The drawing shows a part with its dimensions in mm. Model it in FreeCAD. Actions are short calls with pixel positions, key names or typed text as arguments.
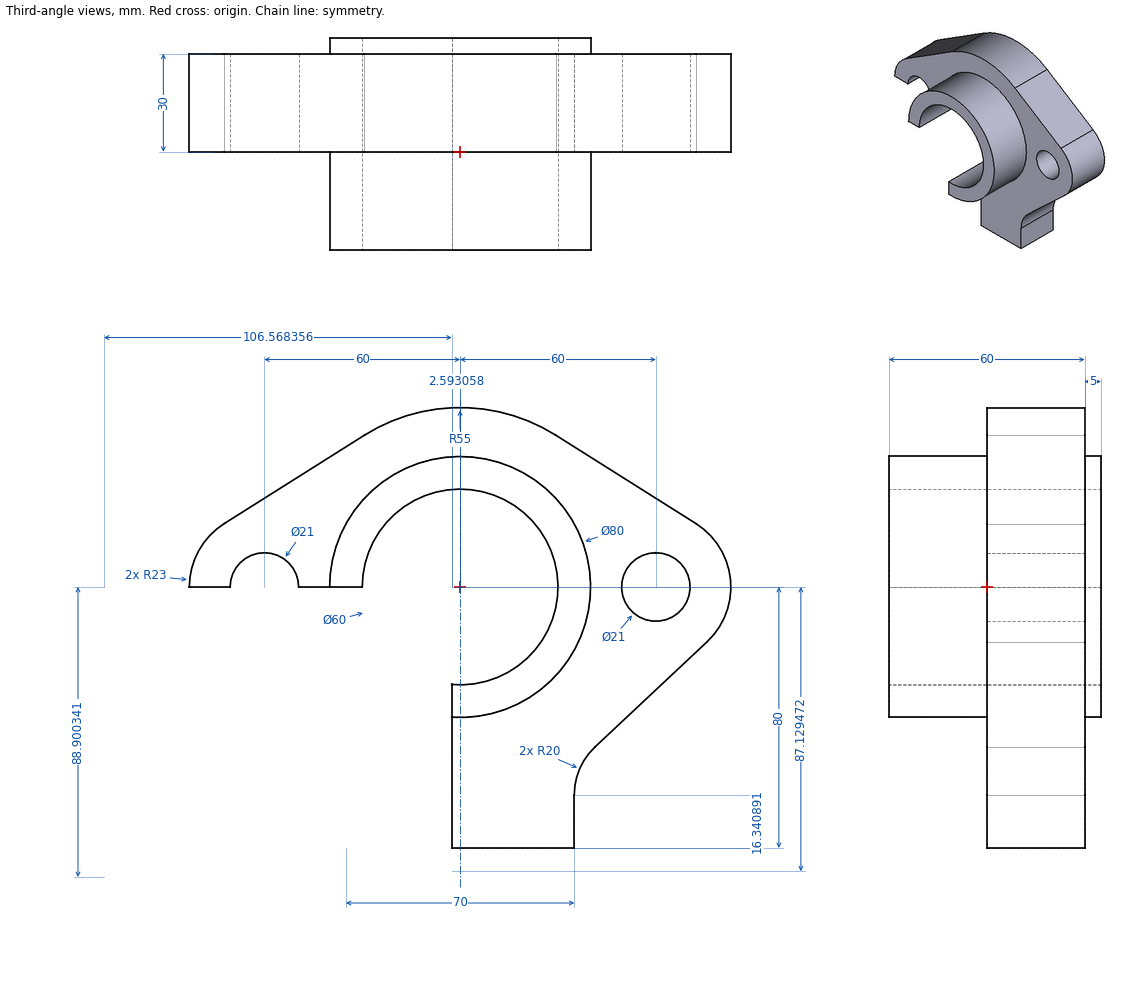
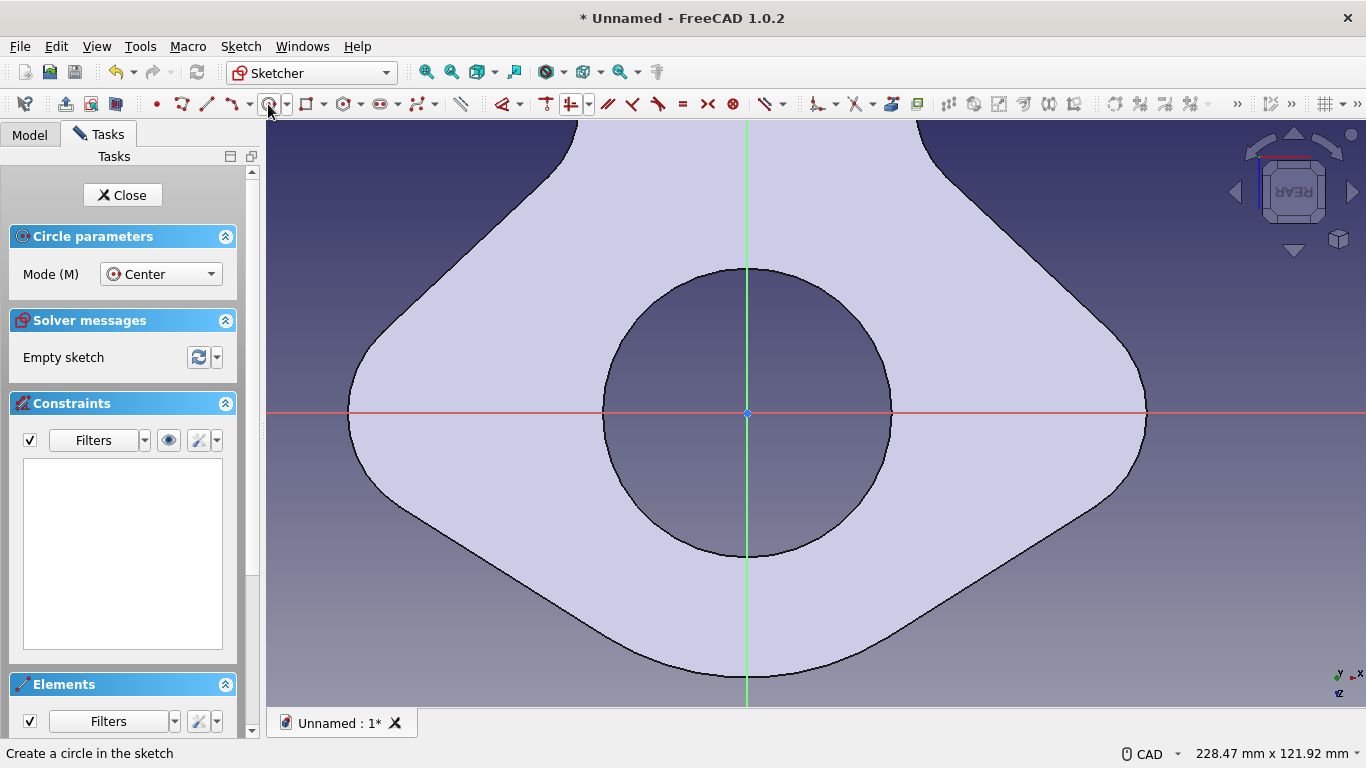
click(747, 413)
move(883, 277)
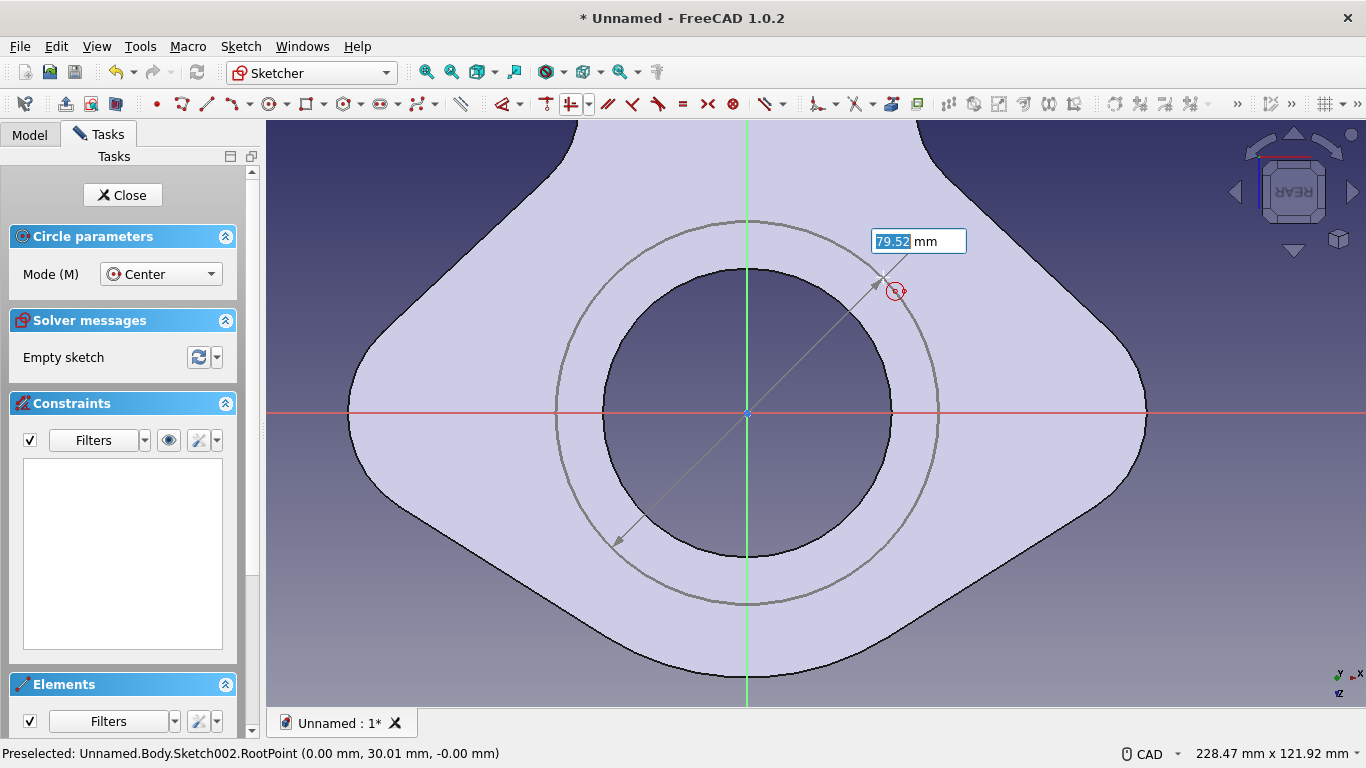
text(80)
key(Return)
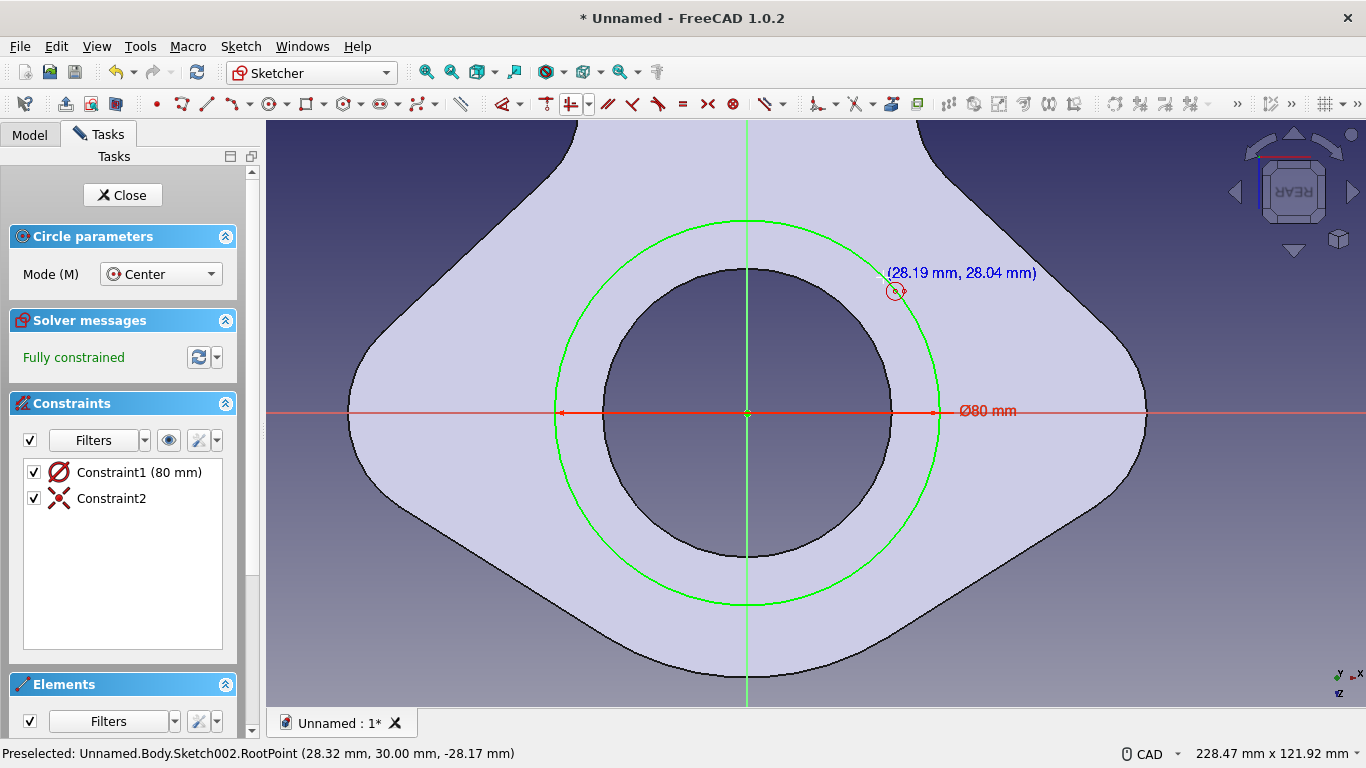
click(747, 413)
move(849, 311)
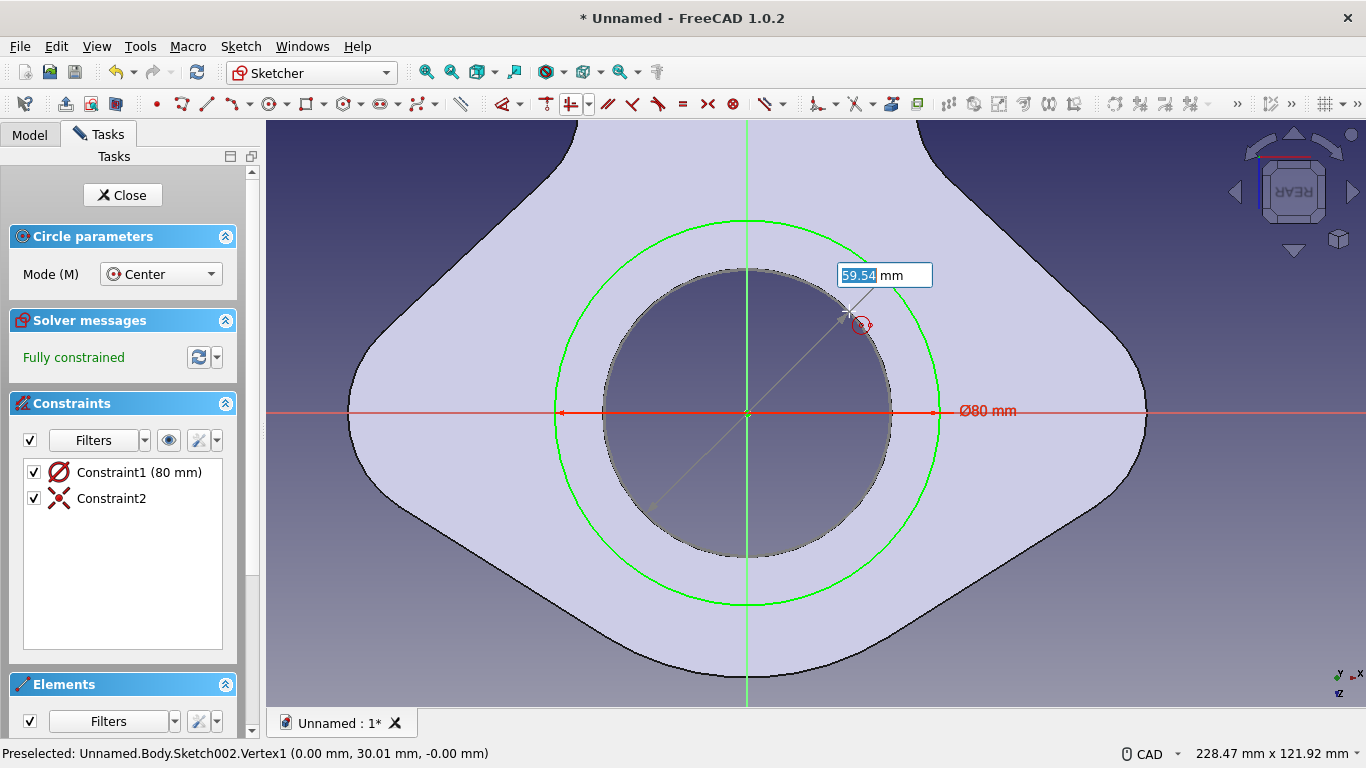
text(60)
key(Return)
key(Escape)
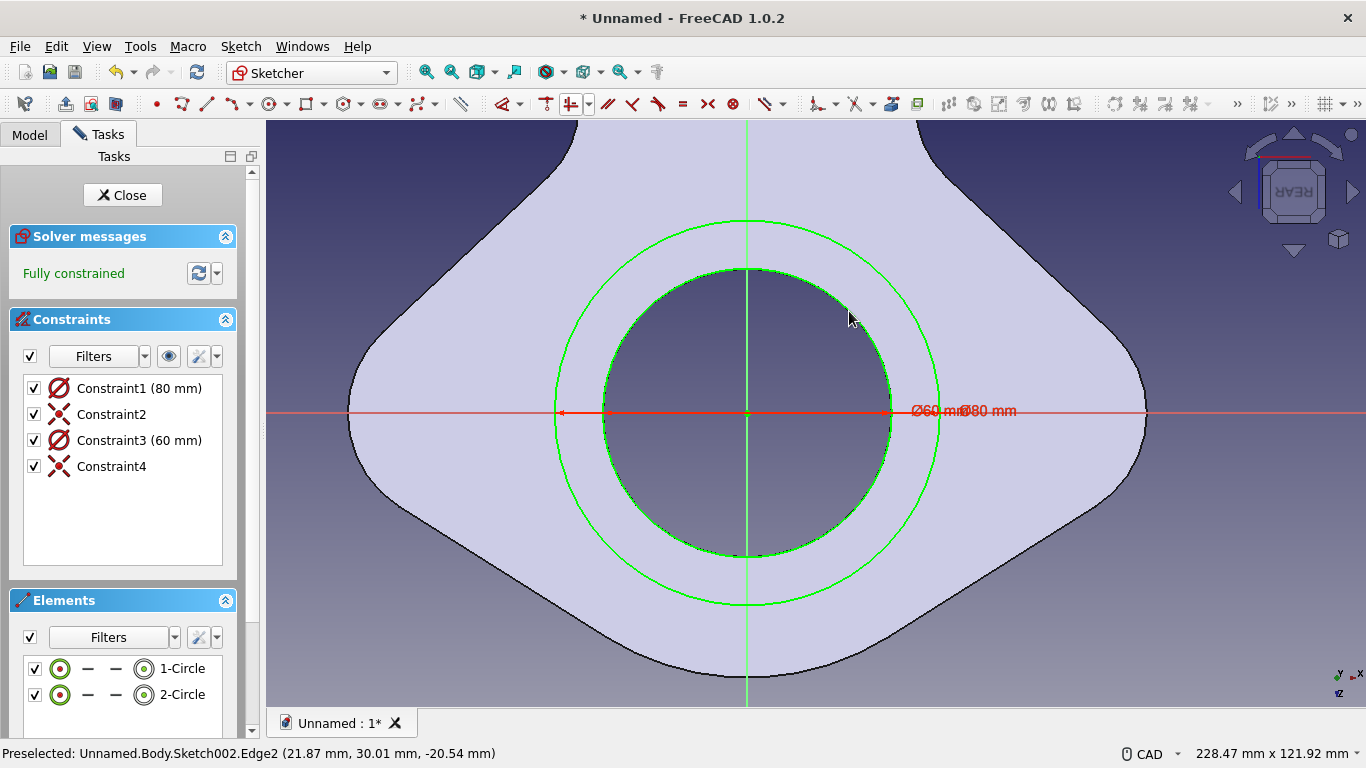
click(123, 195)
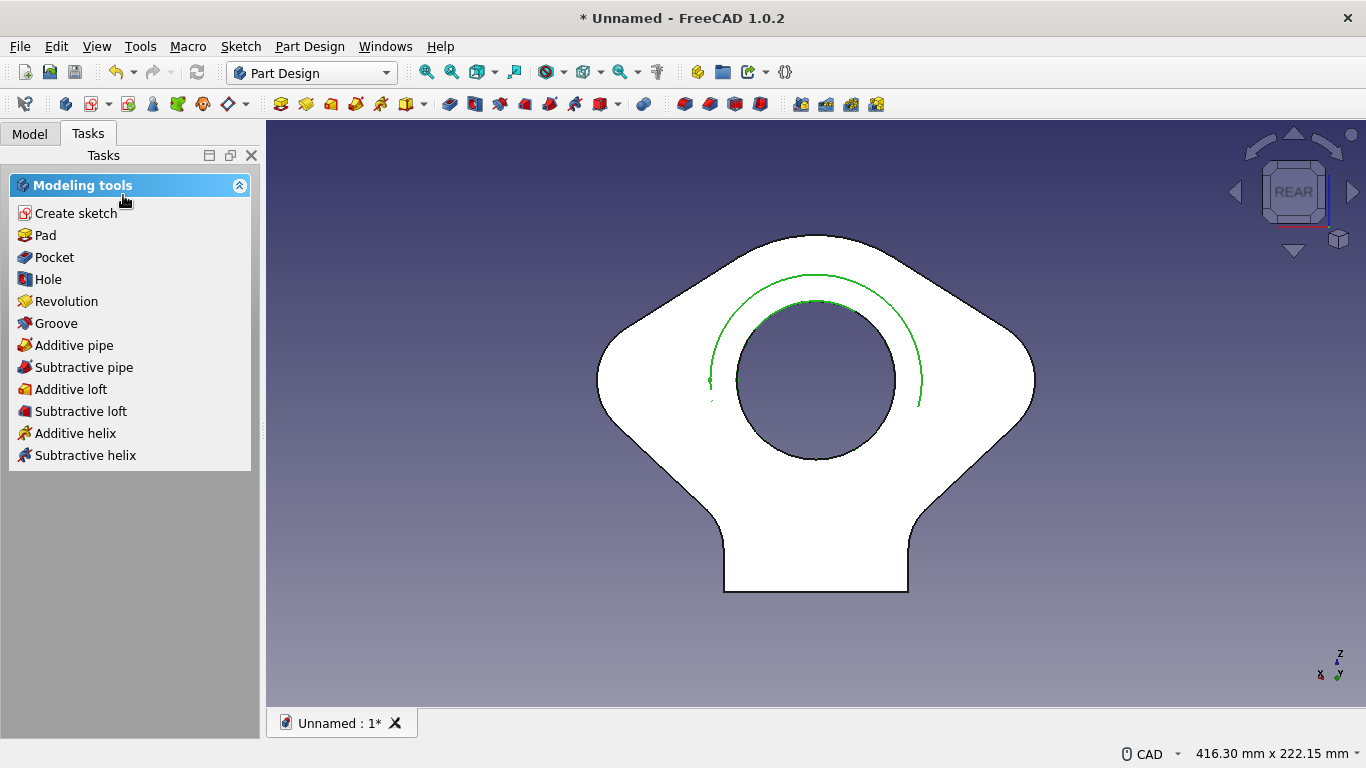
click(281, 104)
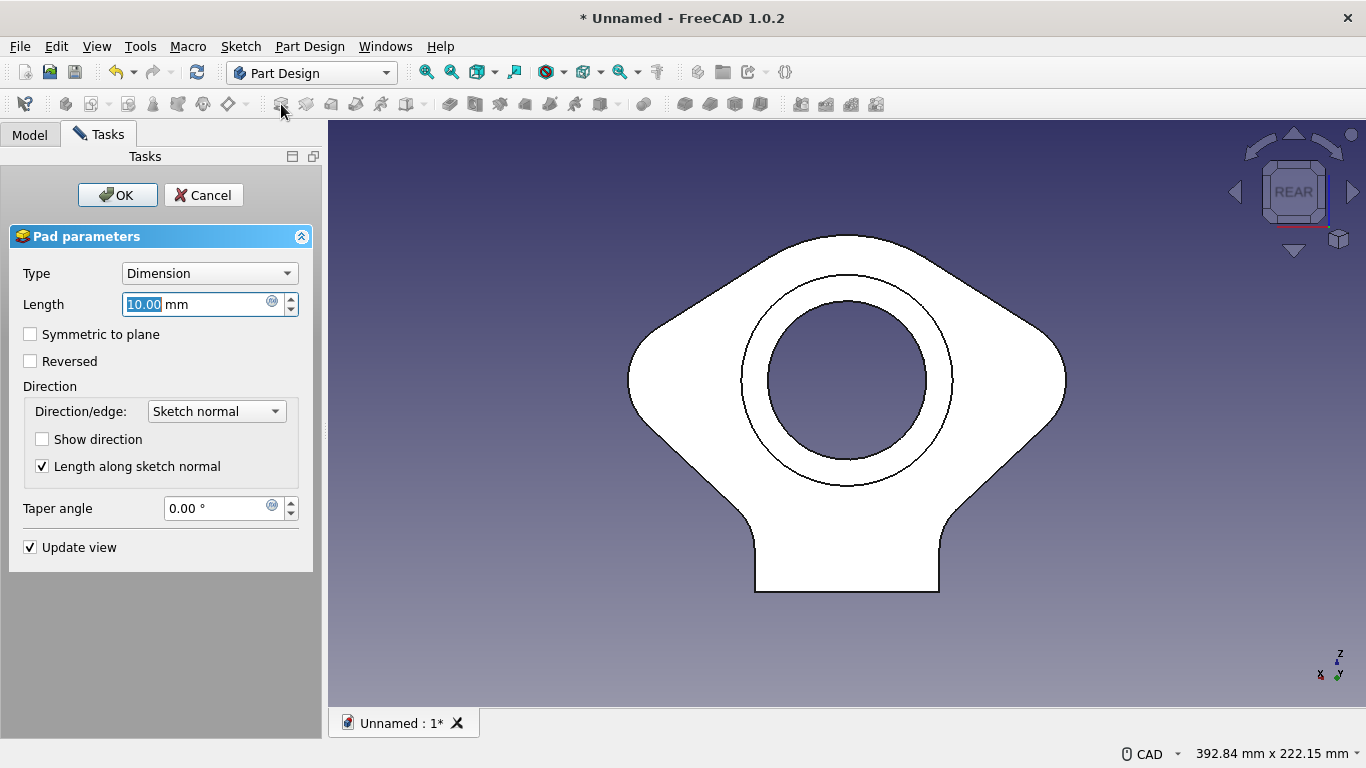
text(5)
key(Tab)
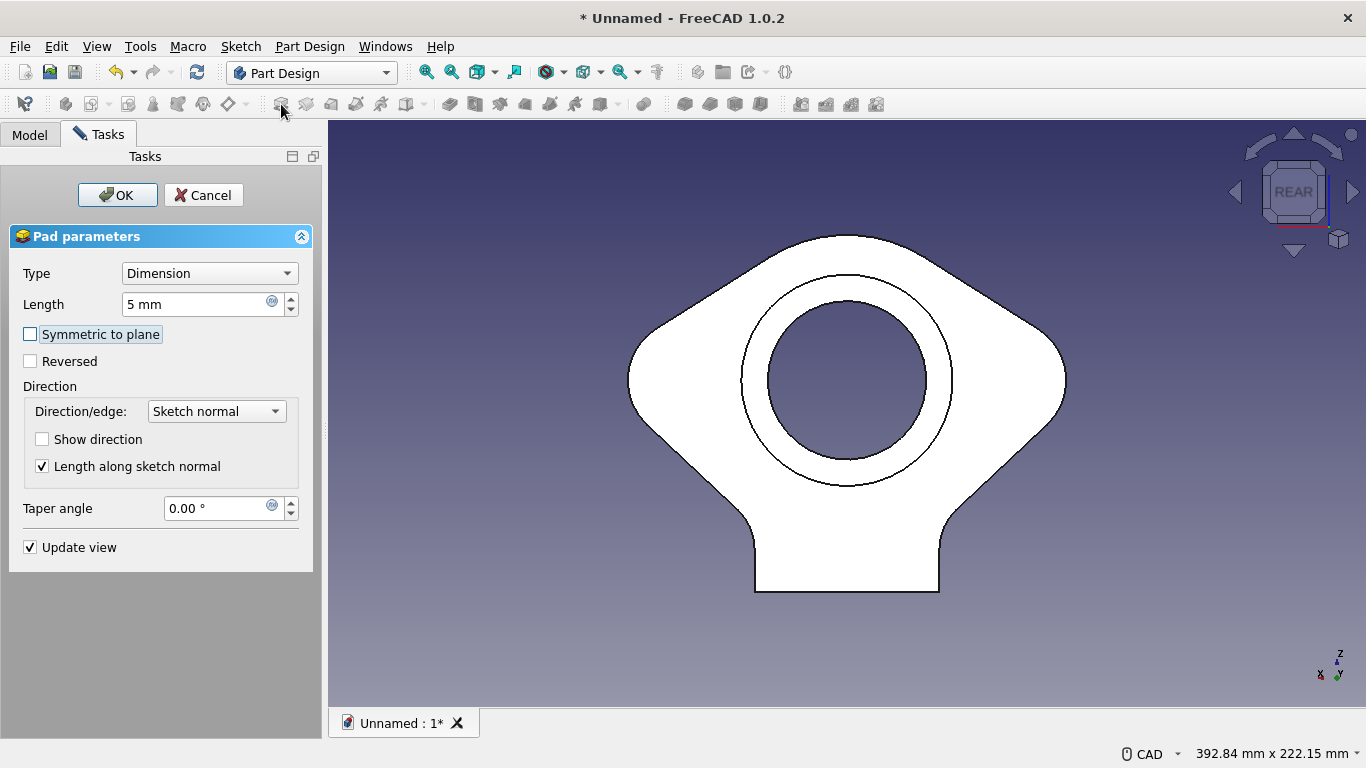
click(118, 195)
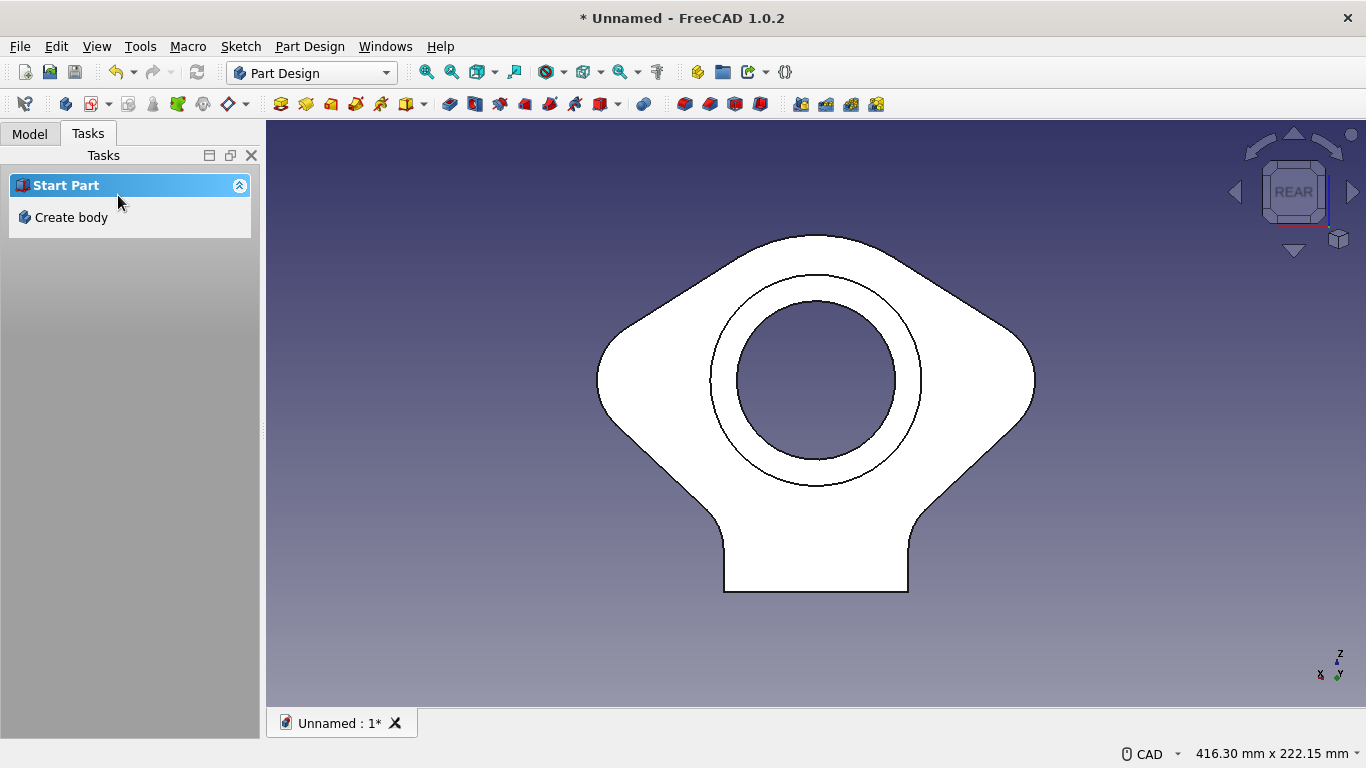
click(90, 104)